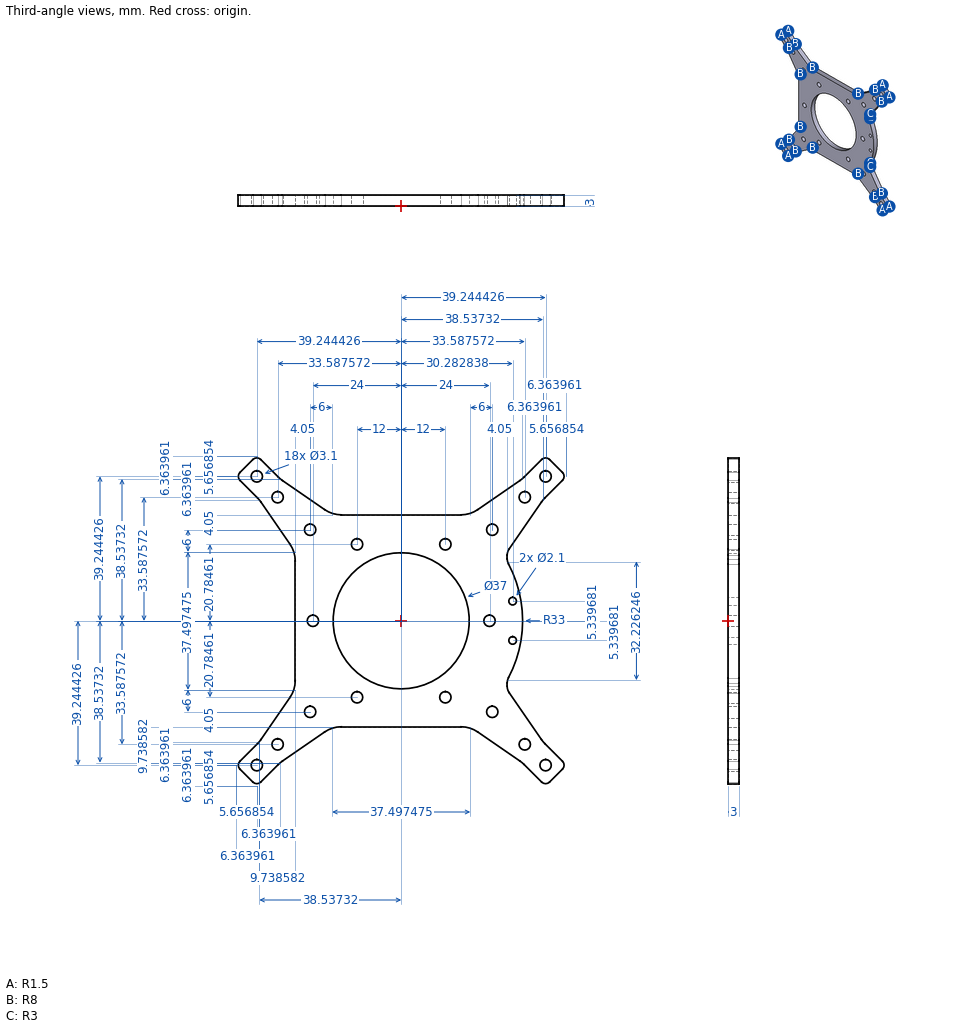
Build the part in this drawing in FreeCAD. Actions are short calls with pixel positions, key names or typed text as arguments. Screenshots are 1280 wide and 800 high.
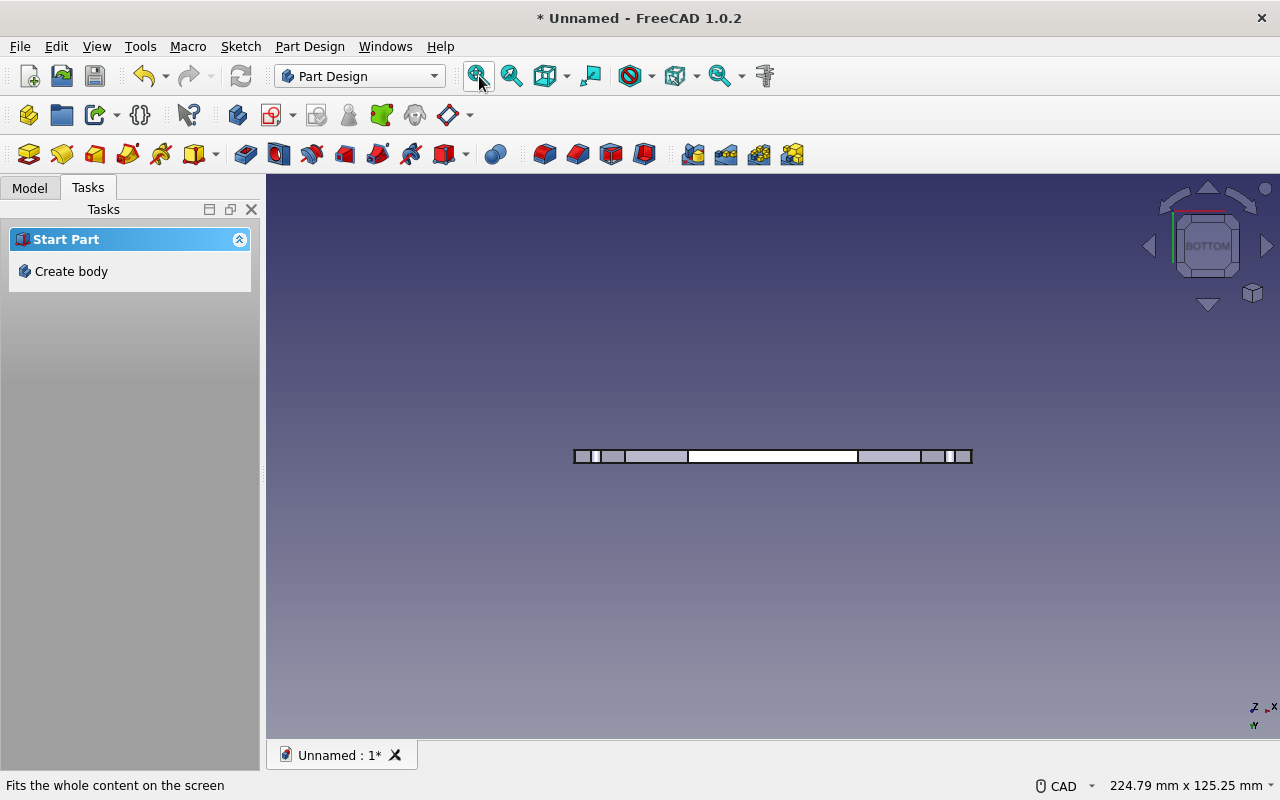
click(479, 76)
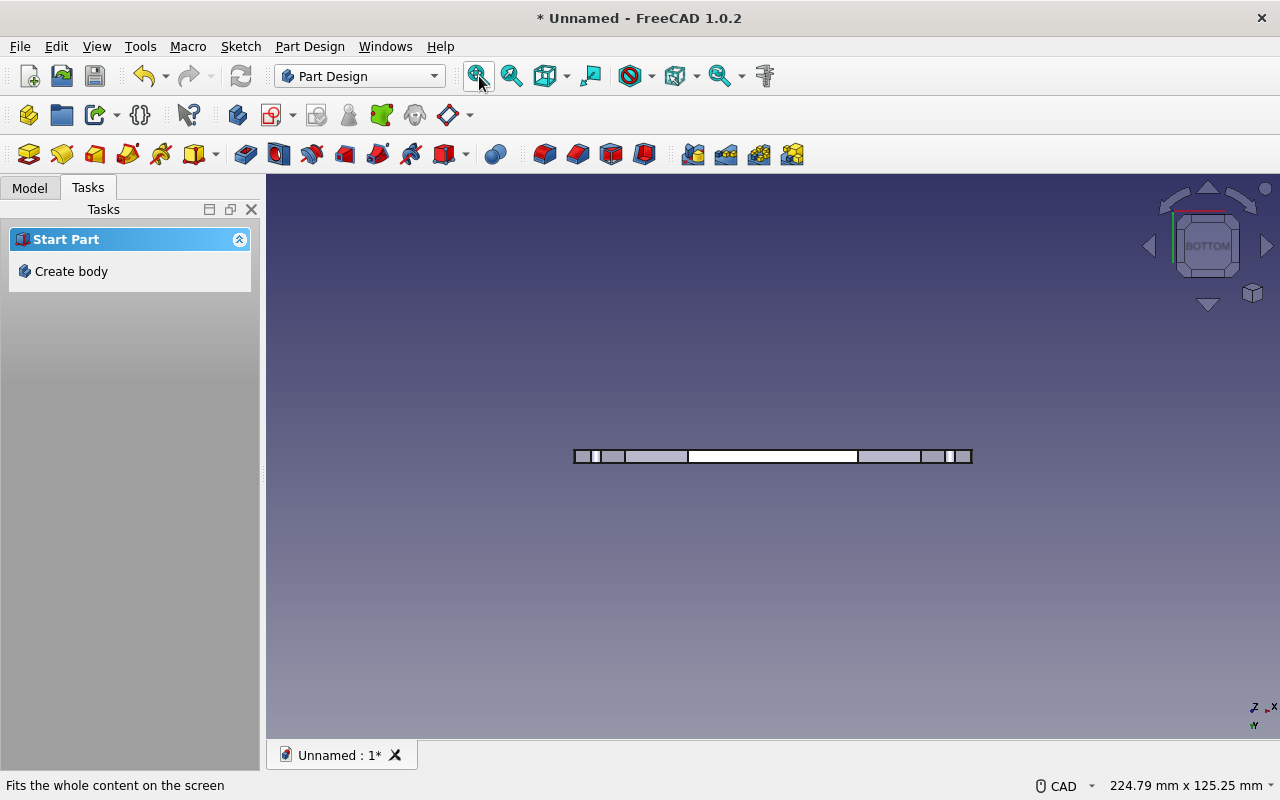
scroll(858, 455, up, 6)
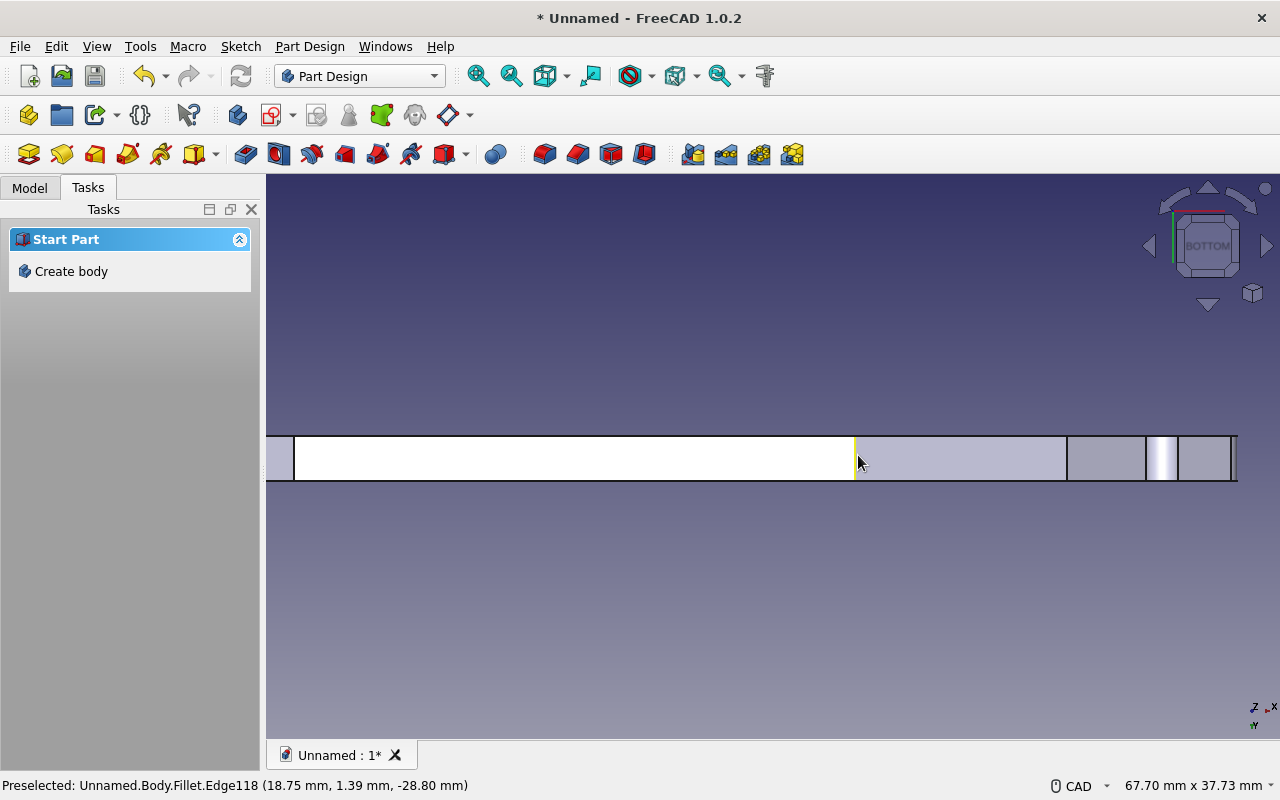
click(479, 76)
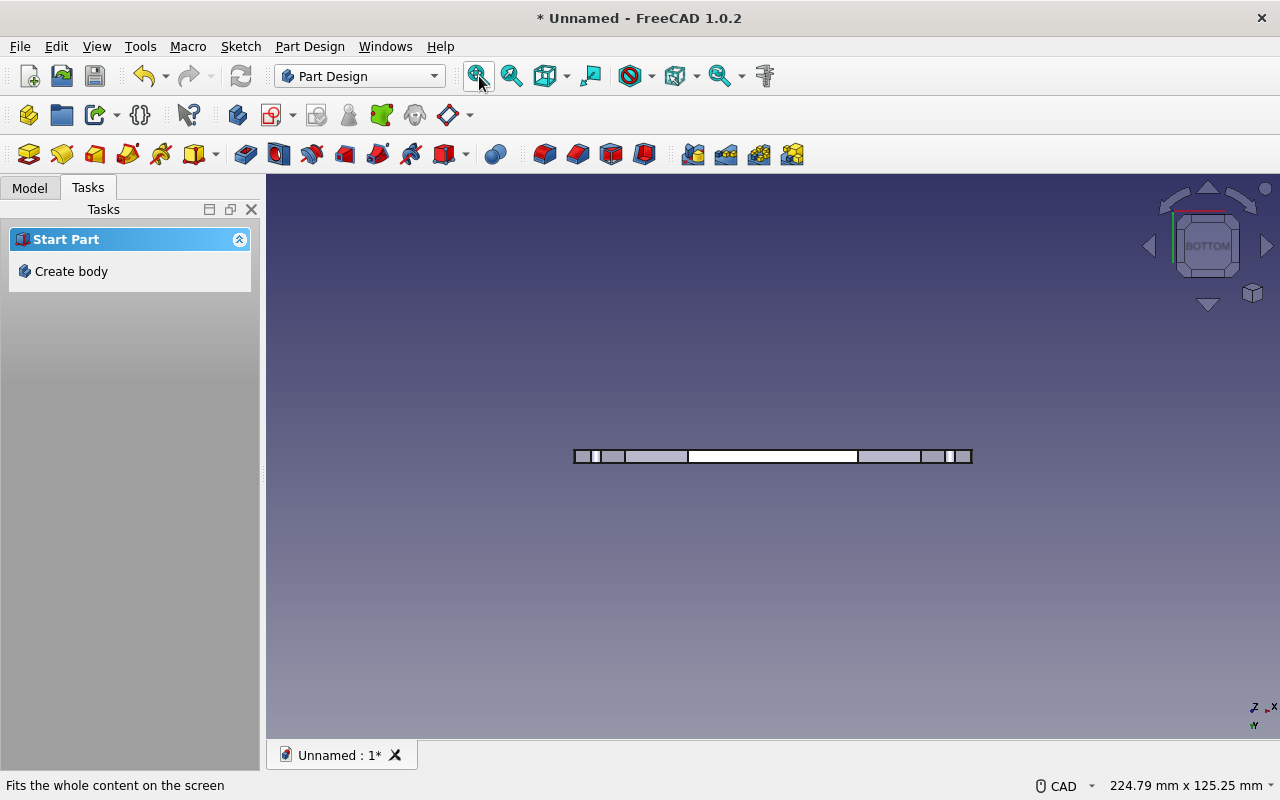
key(4)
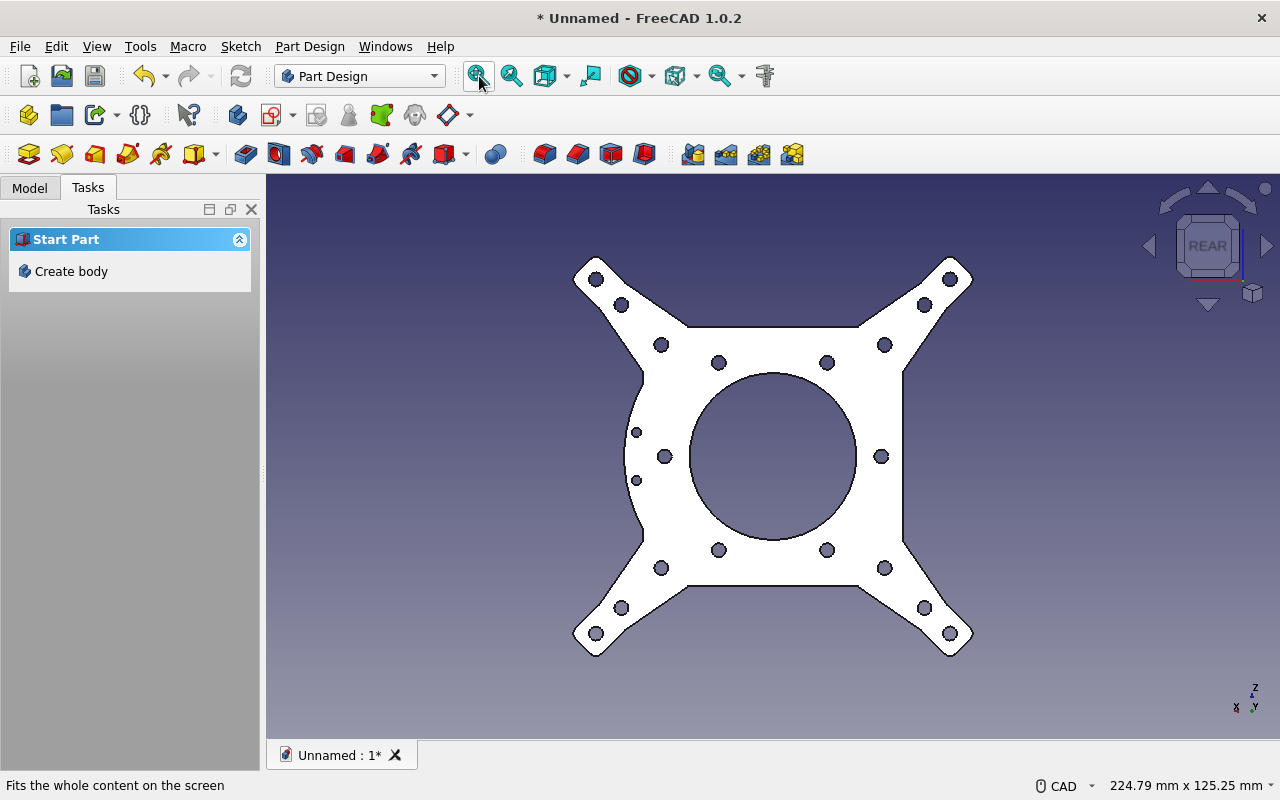
scroll(688, 585, up, 6)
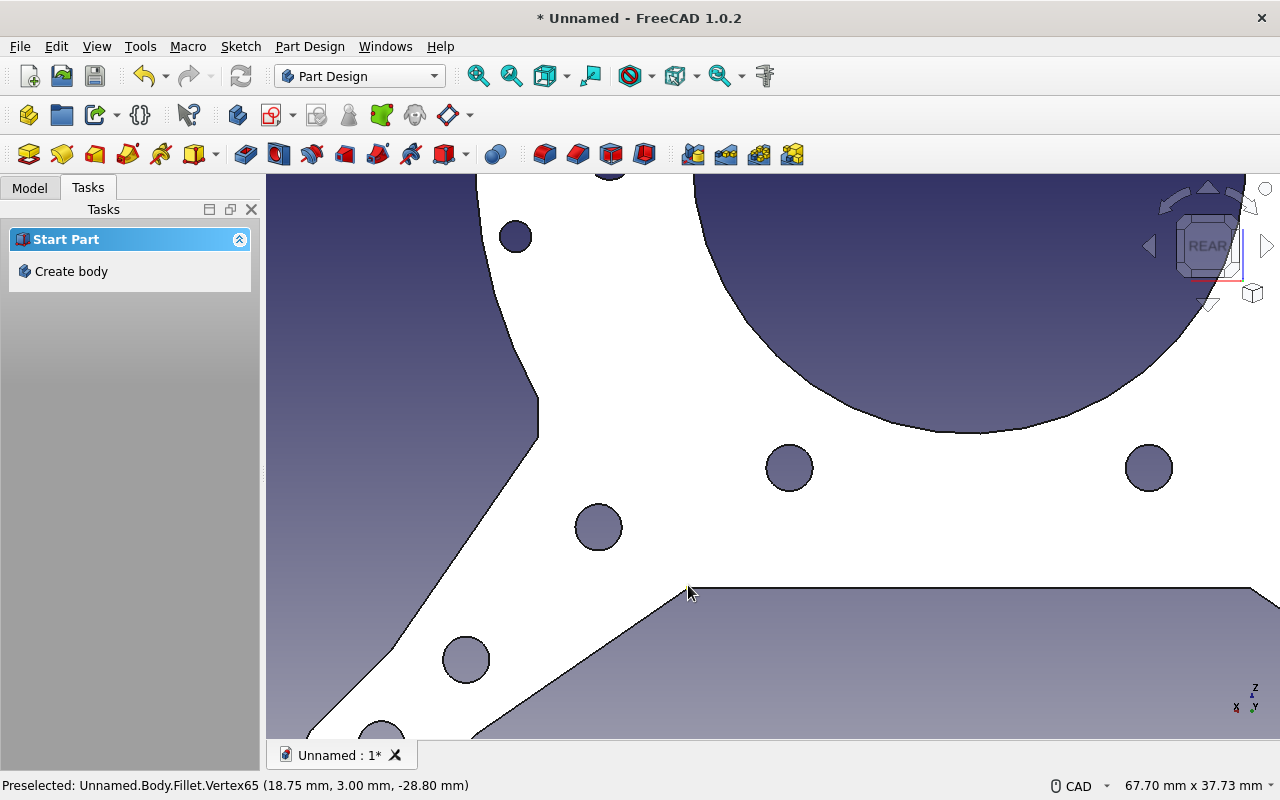
click(479, 76)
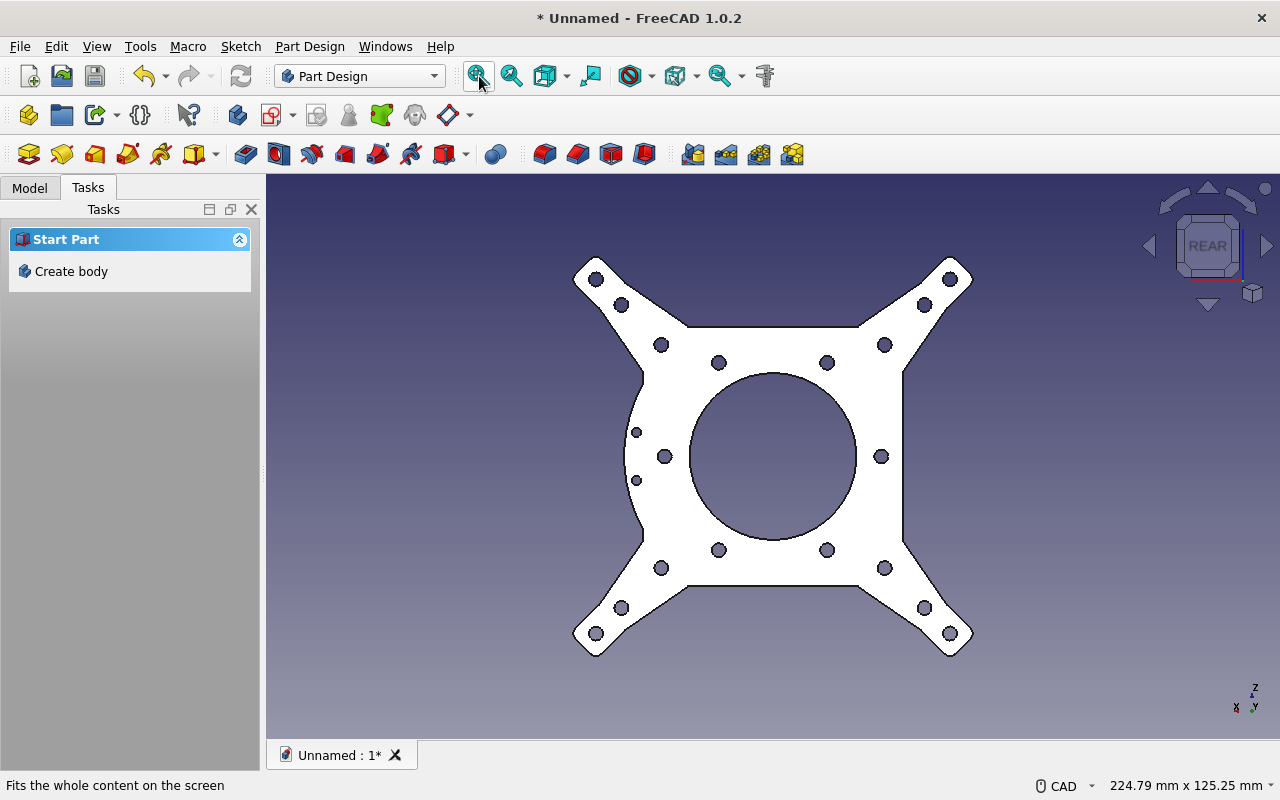
key(6)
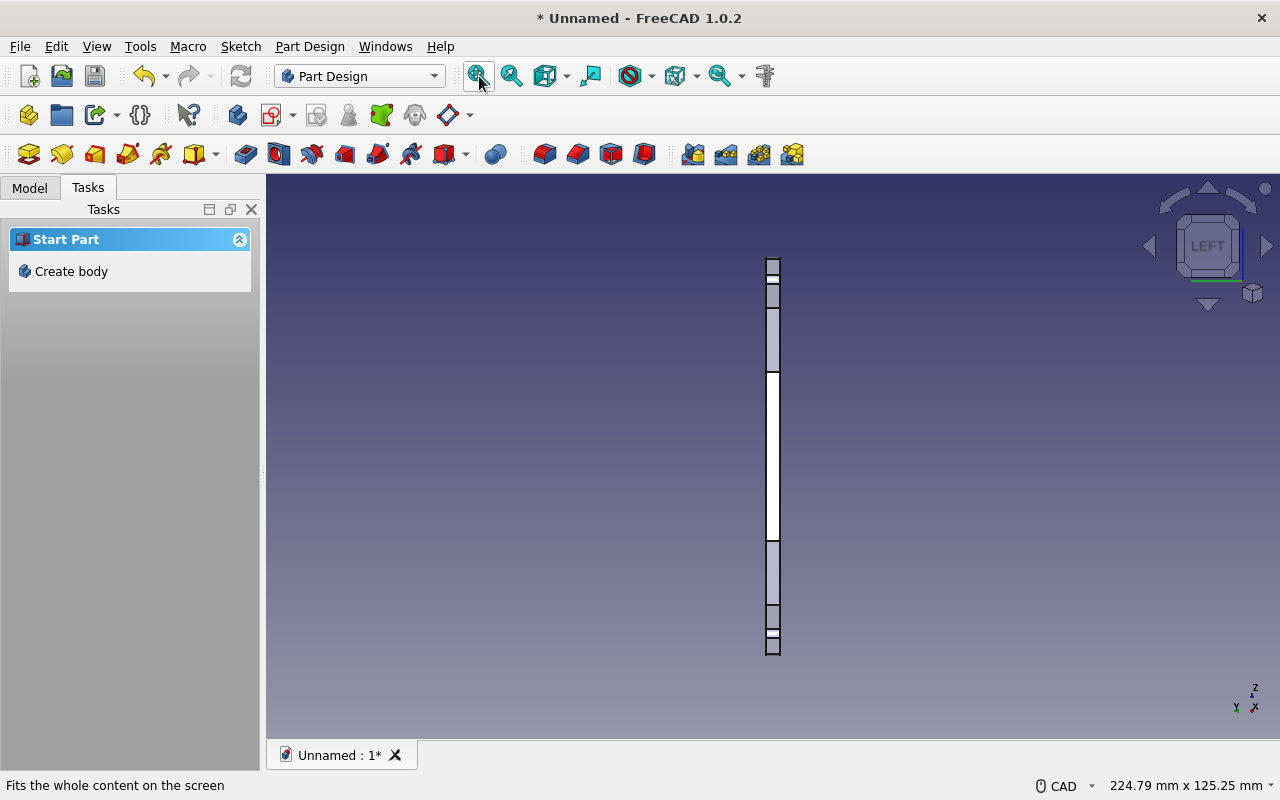
scroll(773, 585, up, 6)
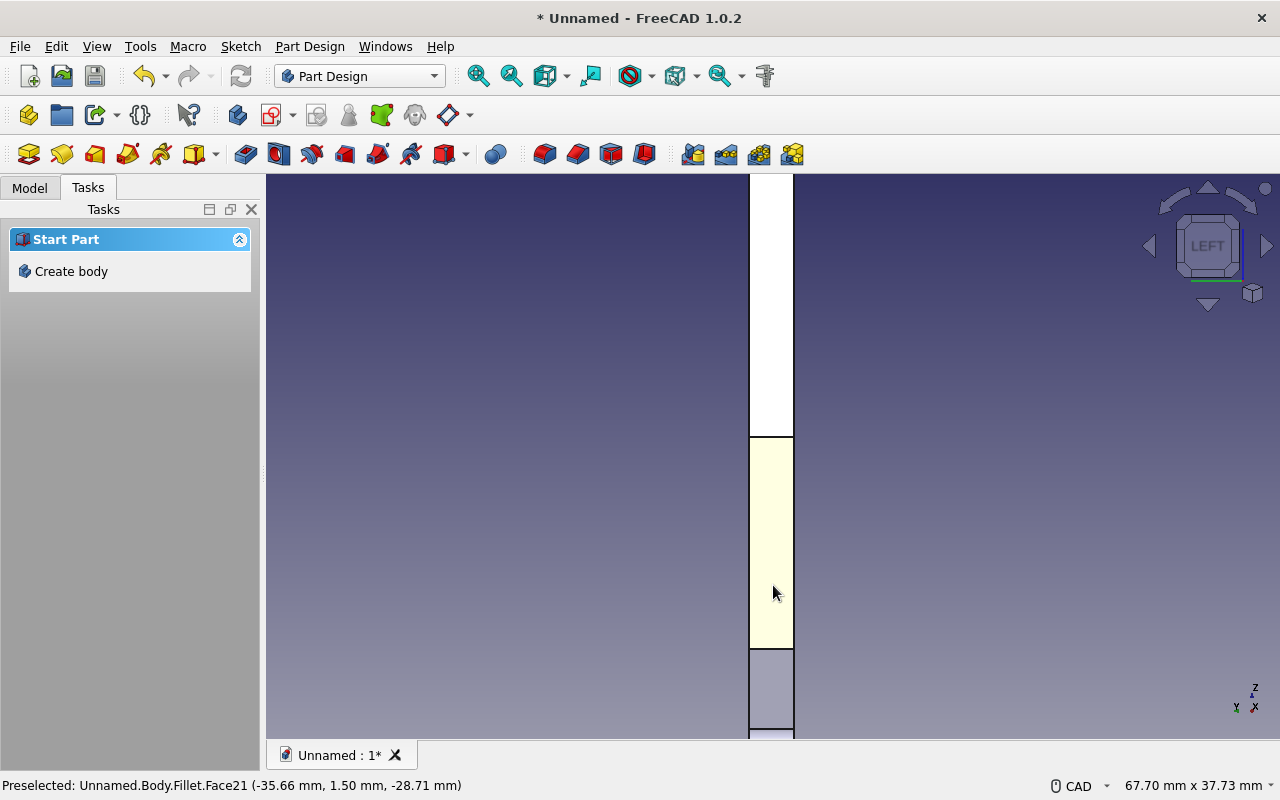
click(479, 76)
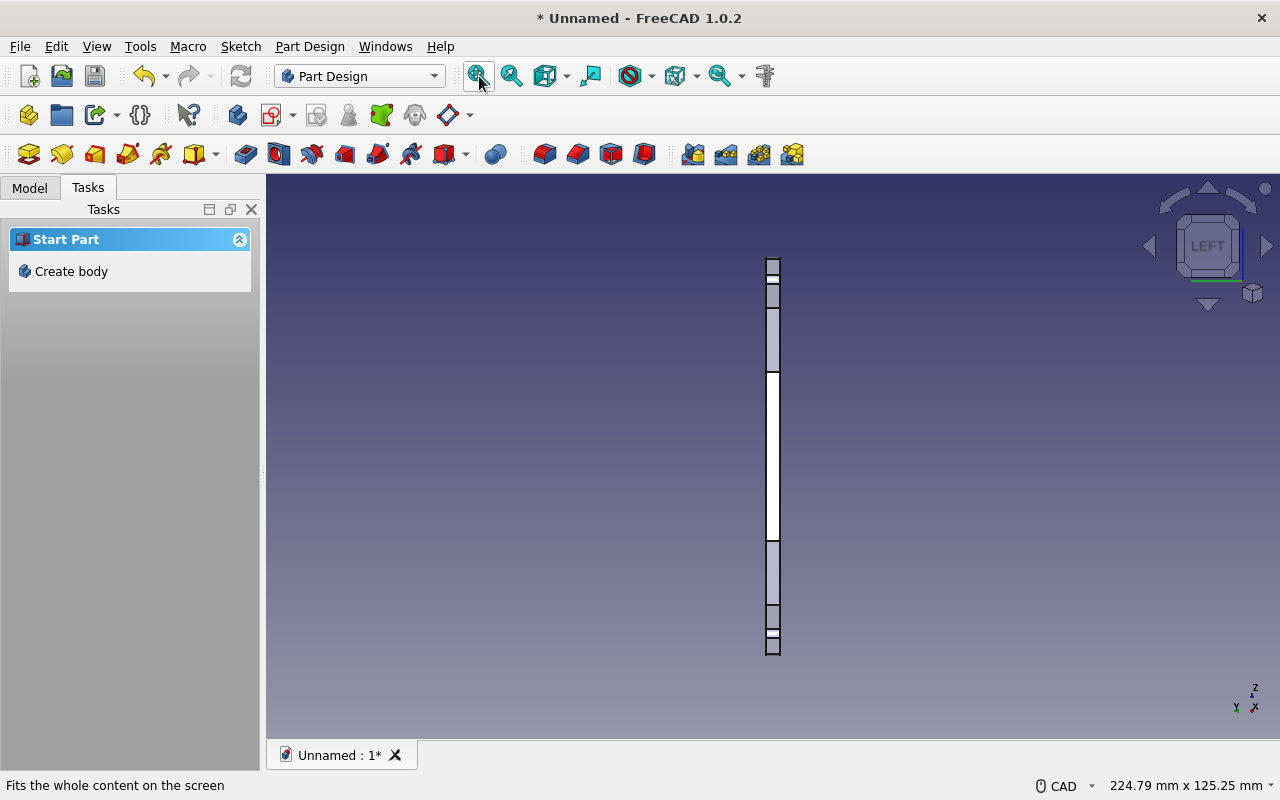
key(v)
key(3)